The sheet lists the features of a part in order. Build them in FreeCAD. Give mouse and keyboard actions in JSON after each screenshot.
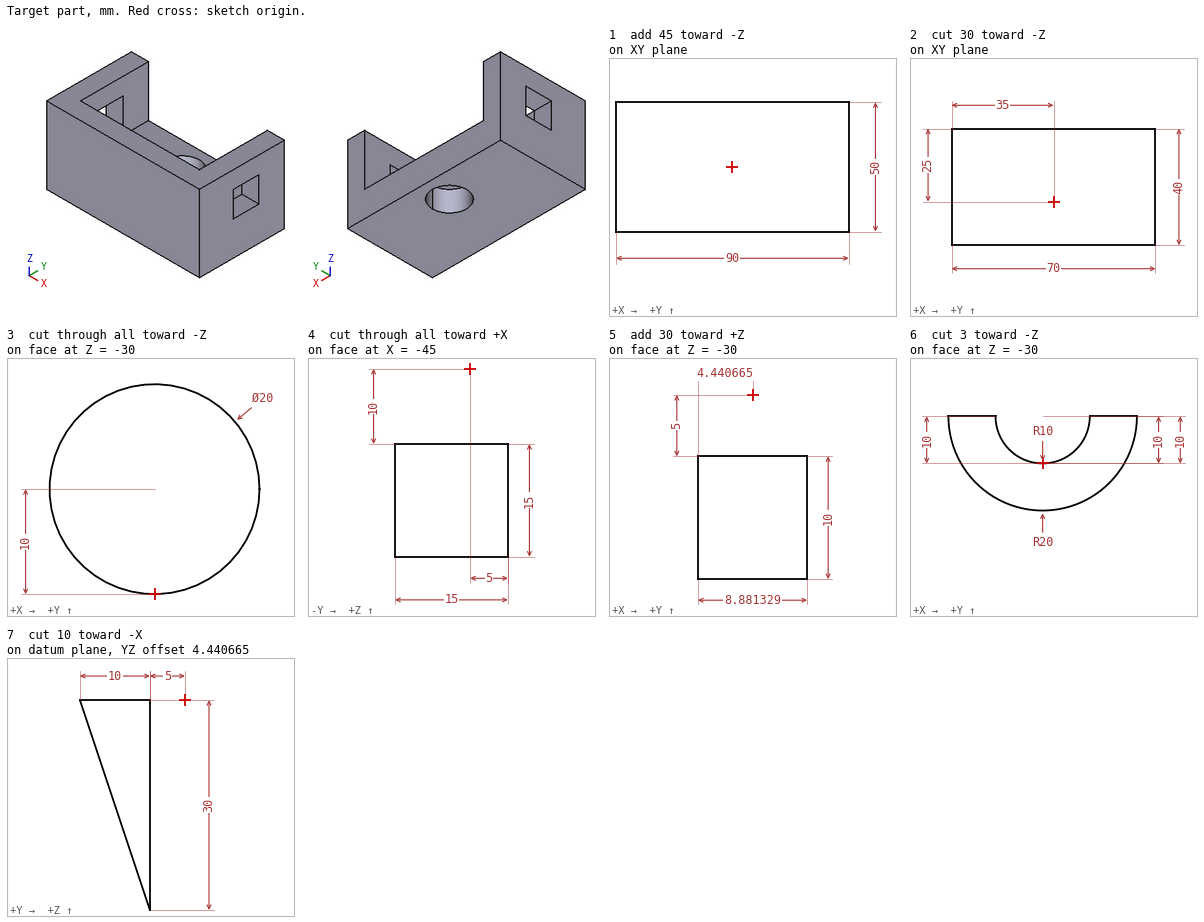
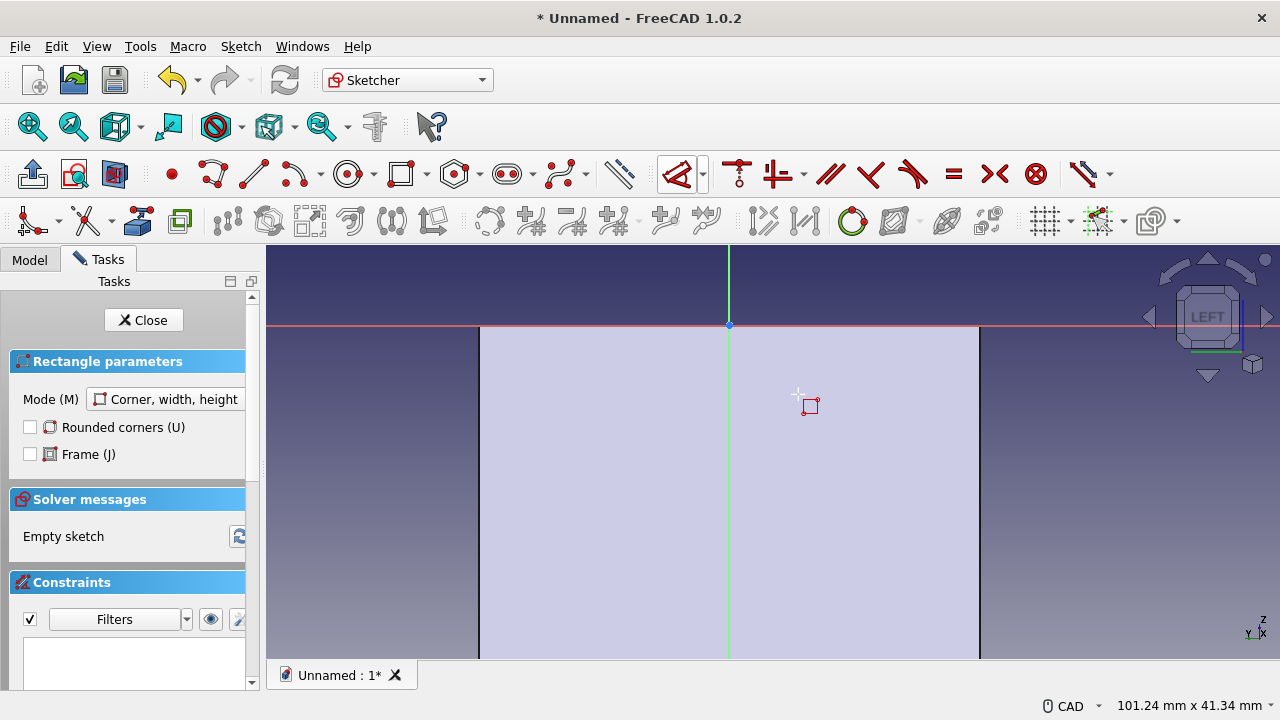
{"action": "left_click", "coordinate": [629, 426]}
{"action": "mouse_move", "coordinate": [779, 576]}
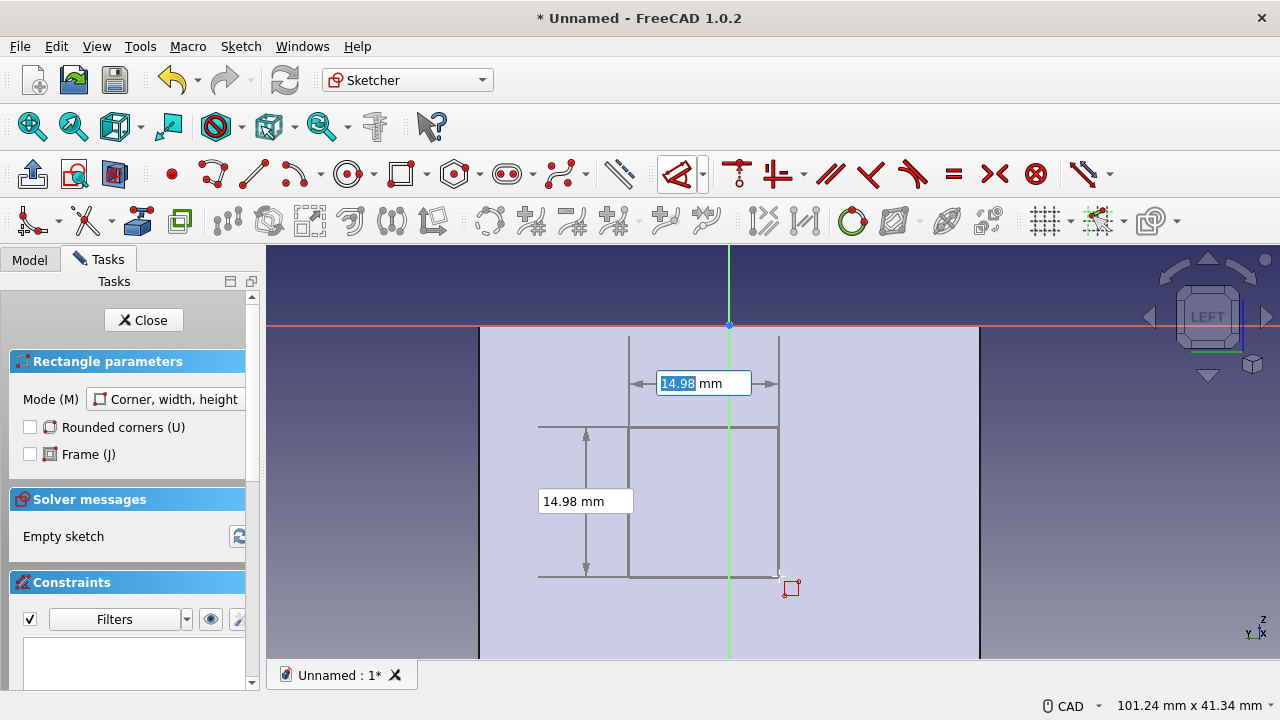
{"action": "type", "text": "15"}
{"action": "key", "text": "Tab"}
{"action": "type", "text": "15"}
{"action": "key", "text": "Return"}
{"action": "key", "text": "Escape"}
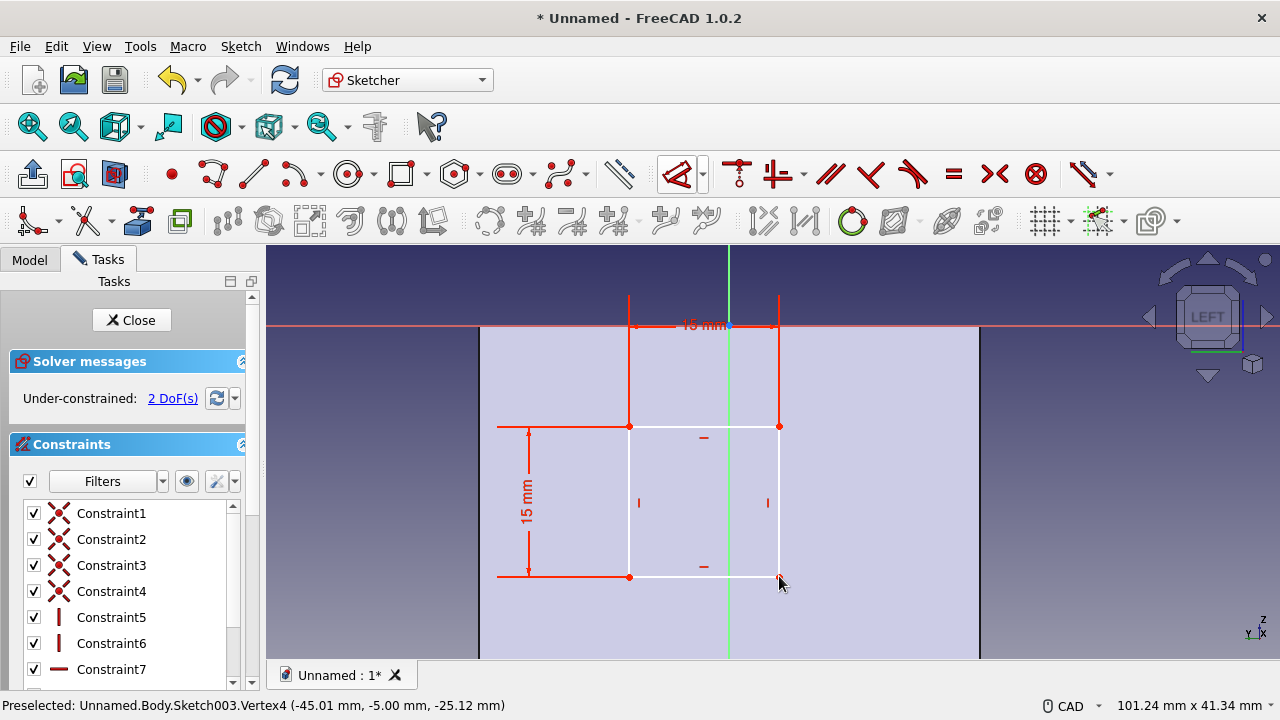
{"action": "left_click", "coordinate": [779, 577]}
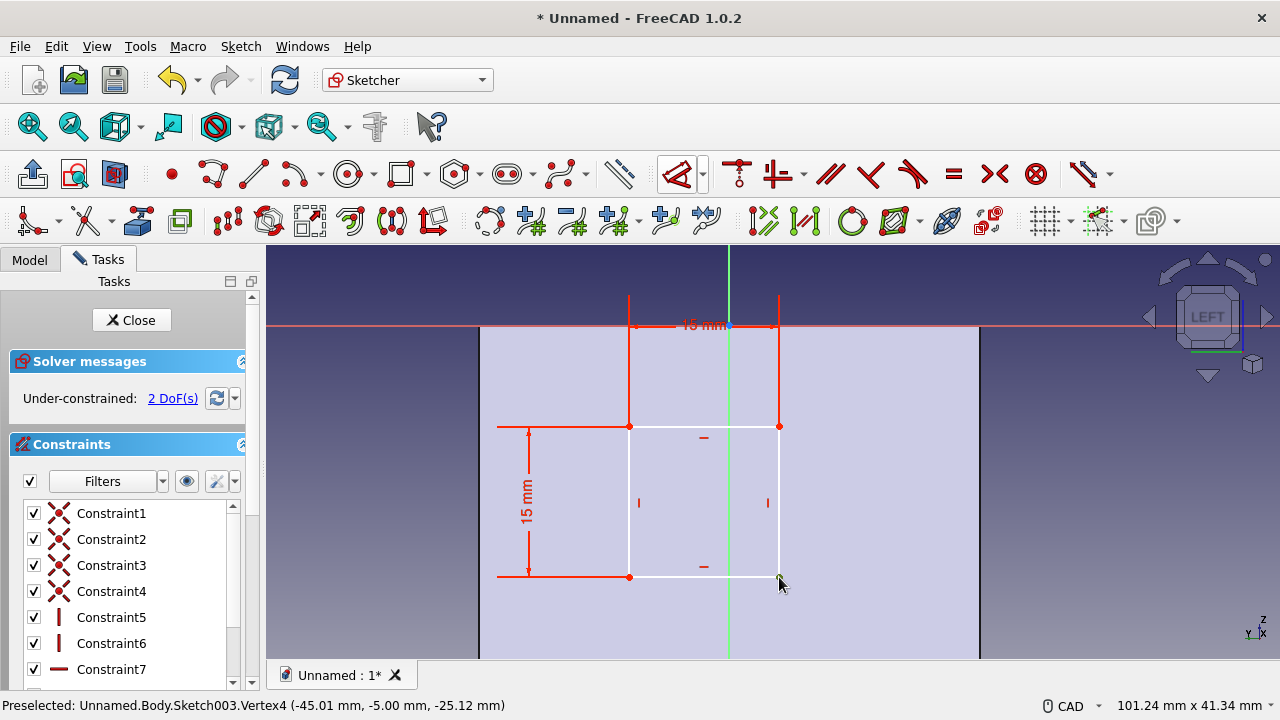
{"action": "key", "text": "l"}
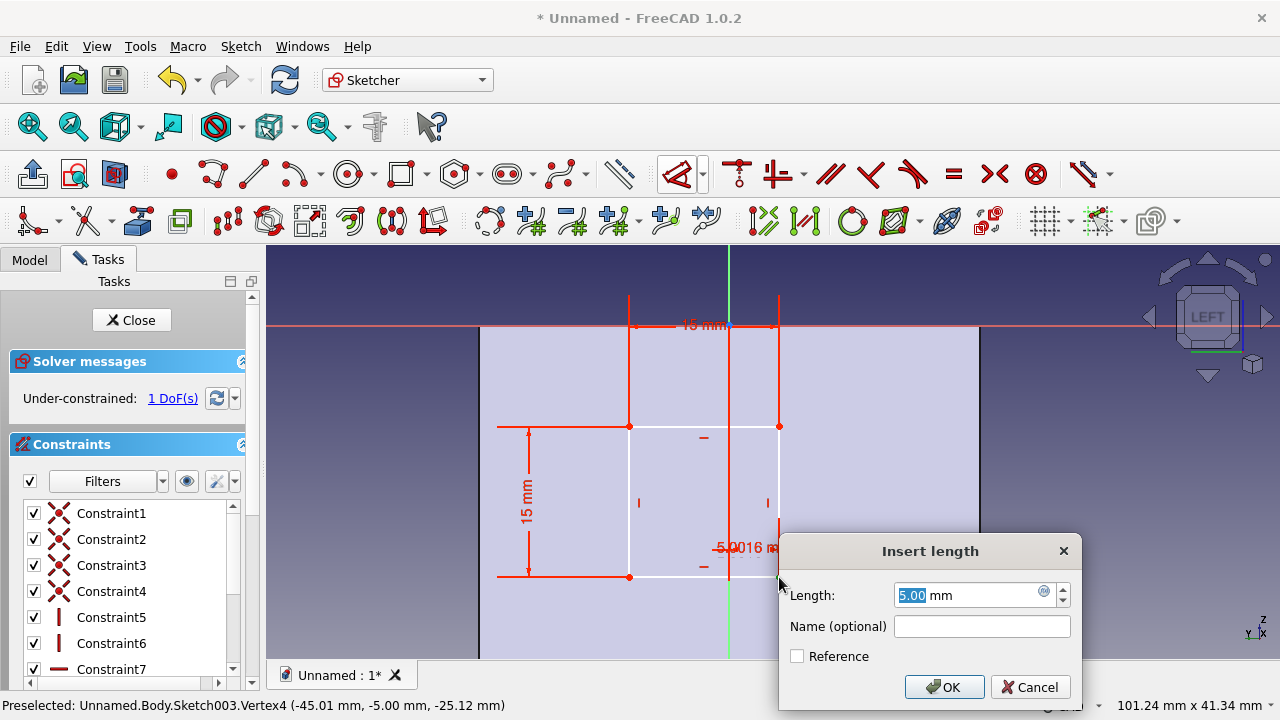
{"action": "type", "text": "5"}
{"action": "key", "text": "Return"}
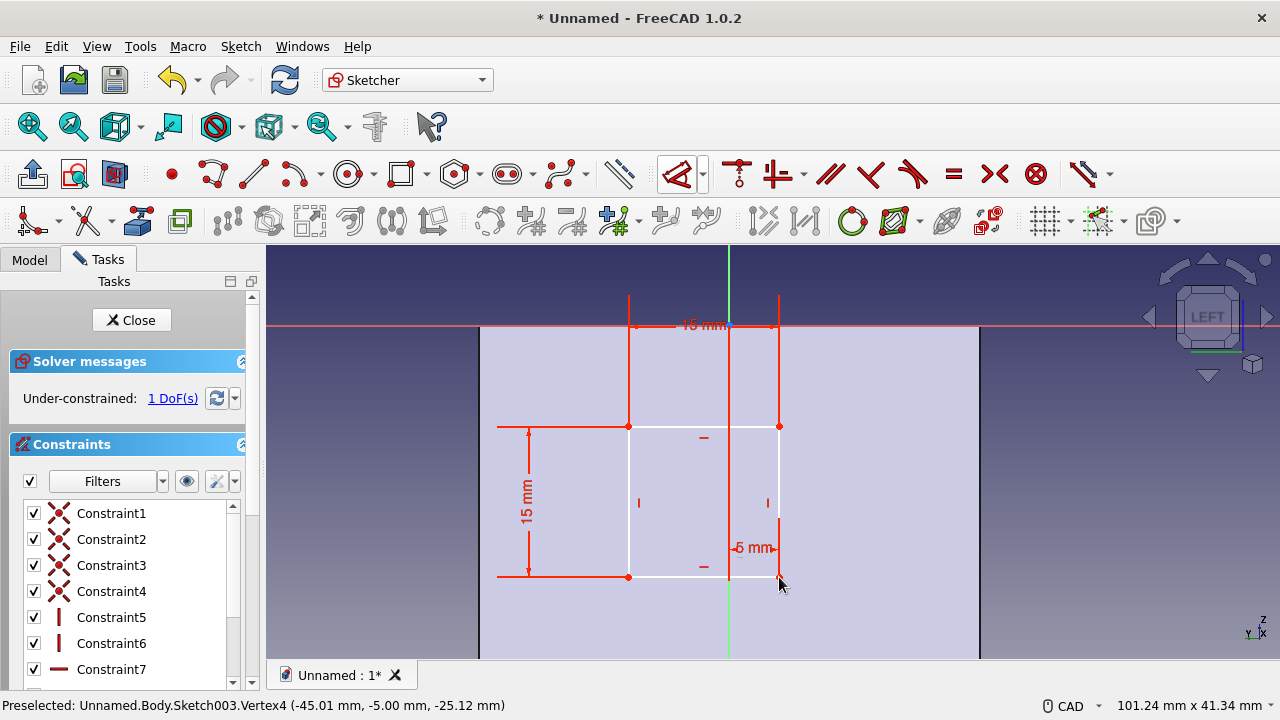
{"action": "left_click", "coordinate": [629, 427]}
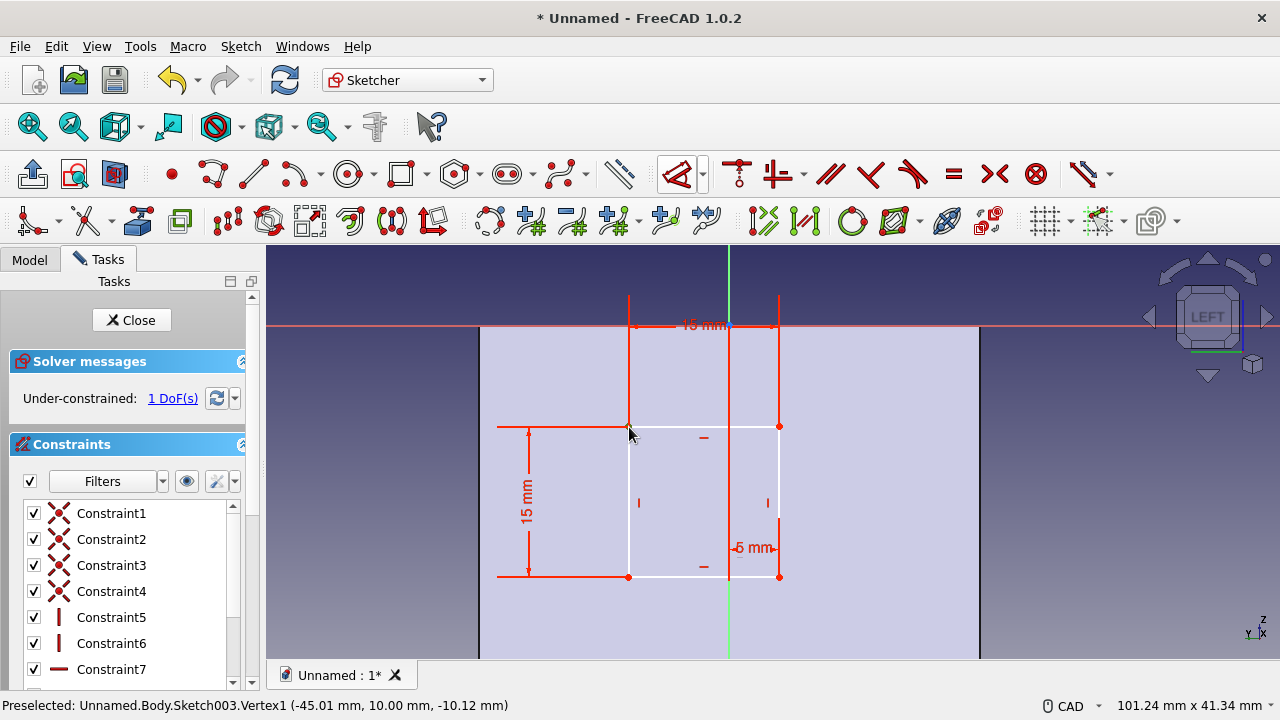
{"action": "key", "text": "i"}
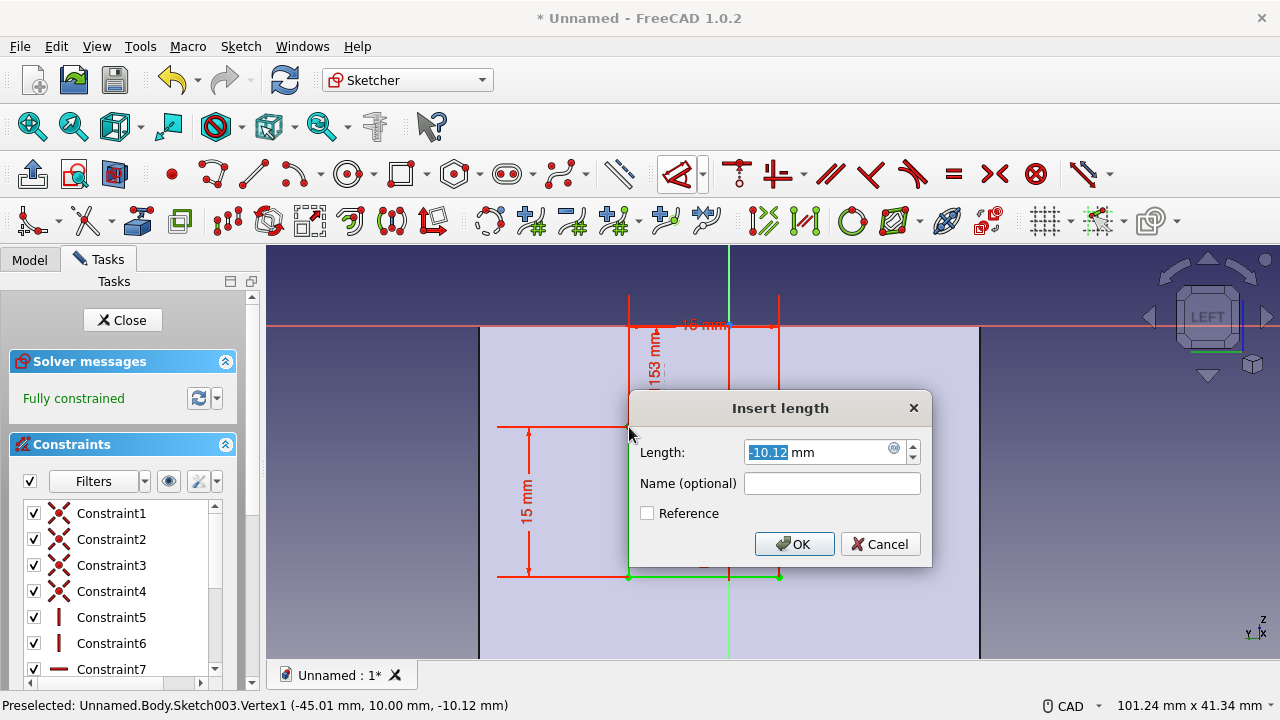
{"action": "type", "text": "-10"}
{"action": "key", "text": "Return"}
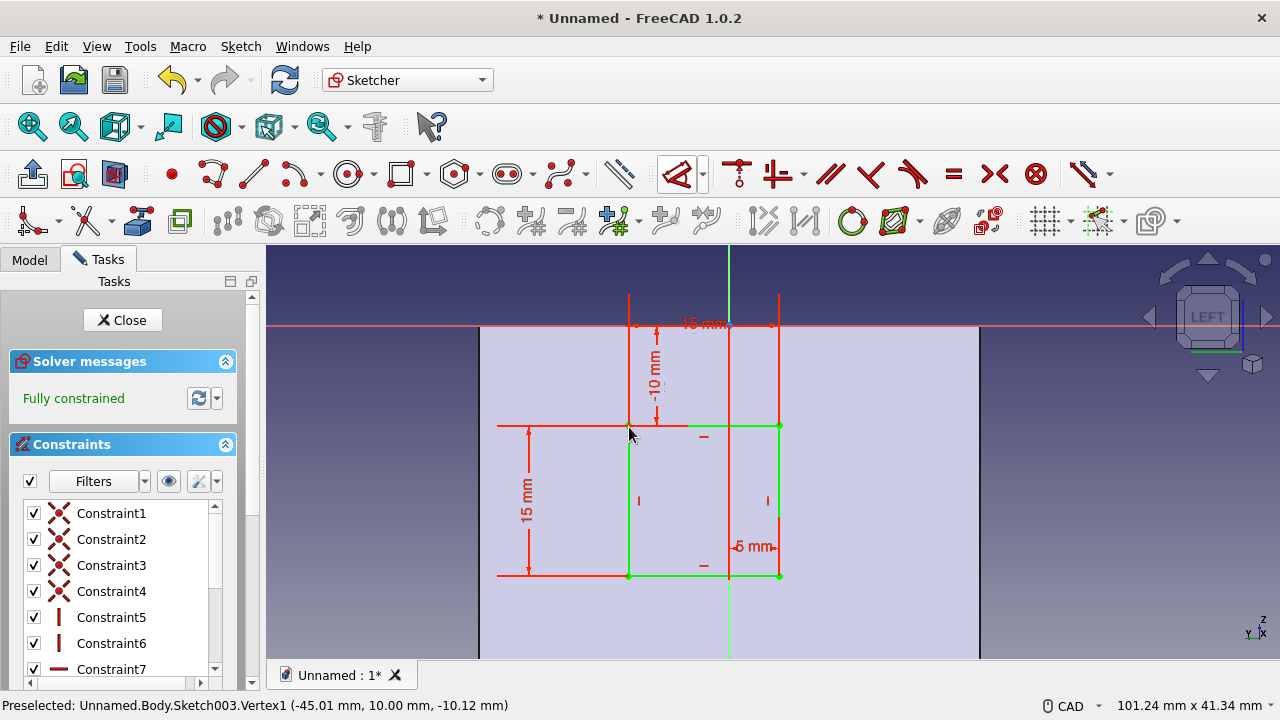
{"action": "left_click", "coordinate": [123, 320]}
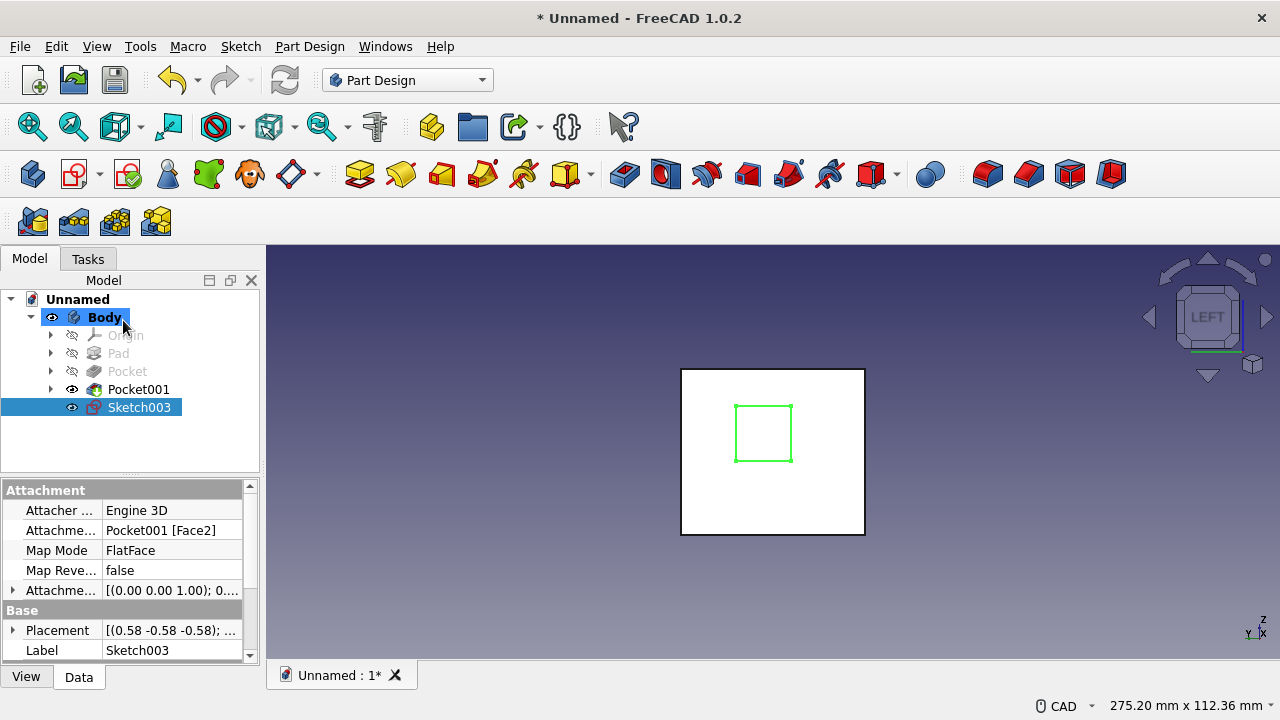
{"action": "left_click", "coordinate": [625, 174]}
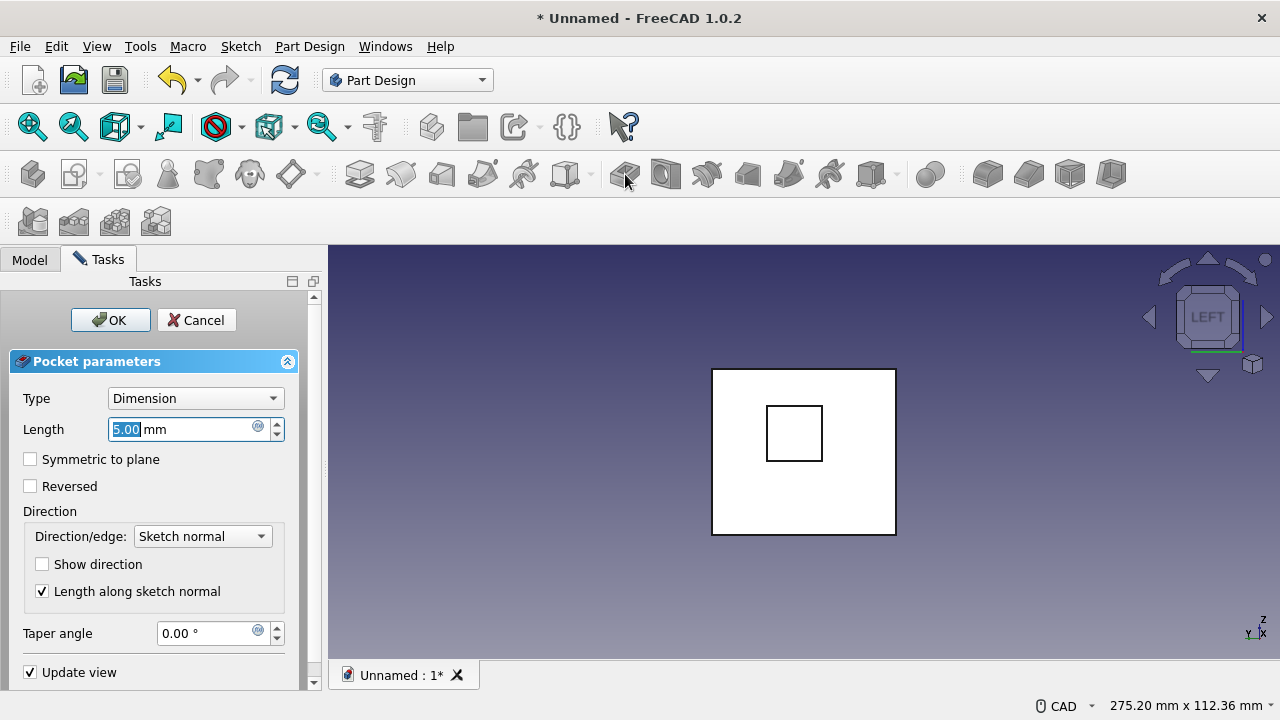
{"action": "left_click", "coordinate": [196, 398]}